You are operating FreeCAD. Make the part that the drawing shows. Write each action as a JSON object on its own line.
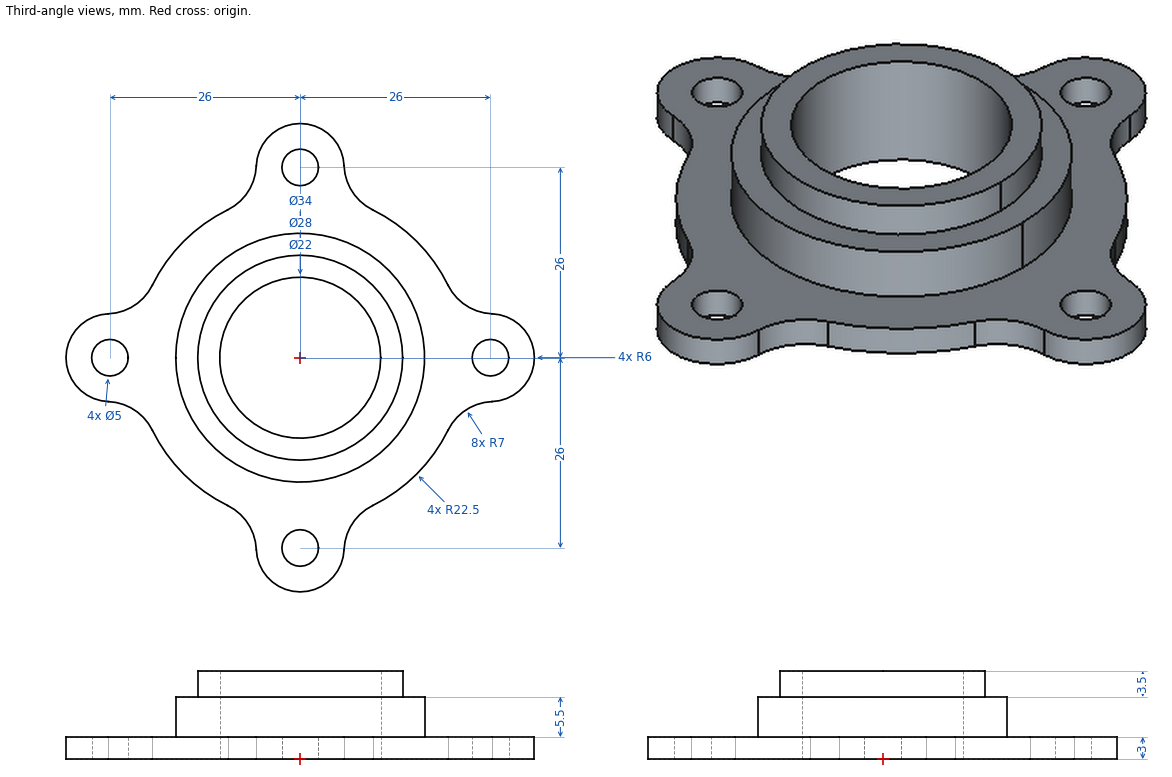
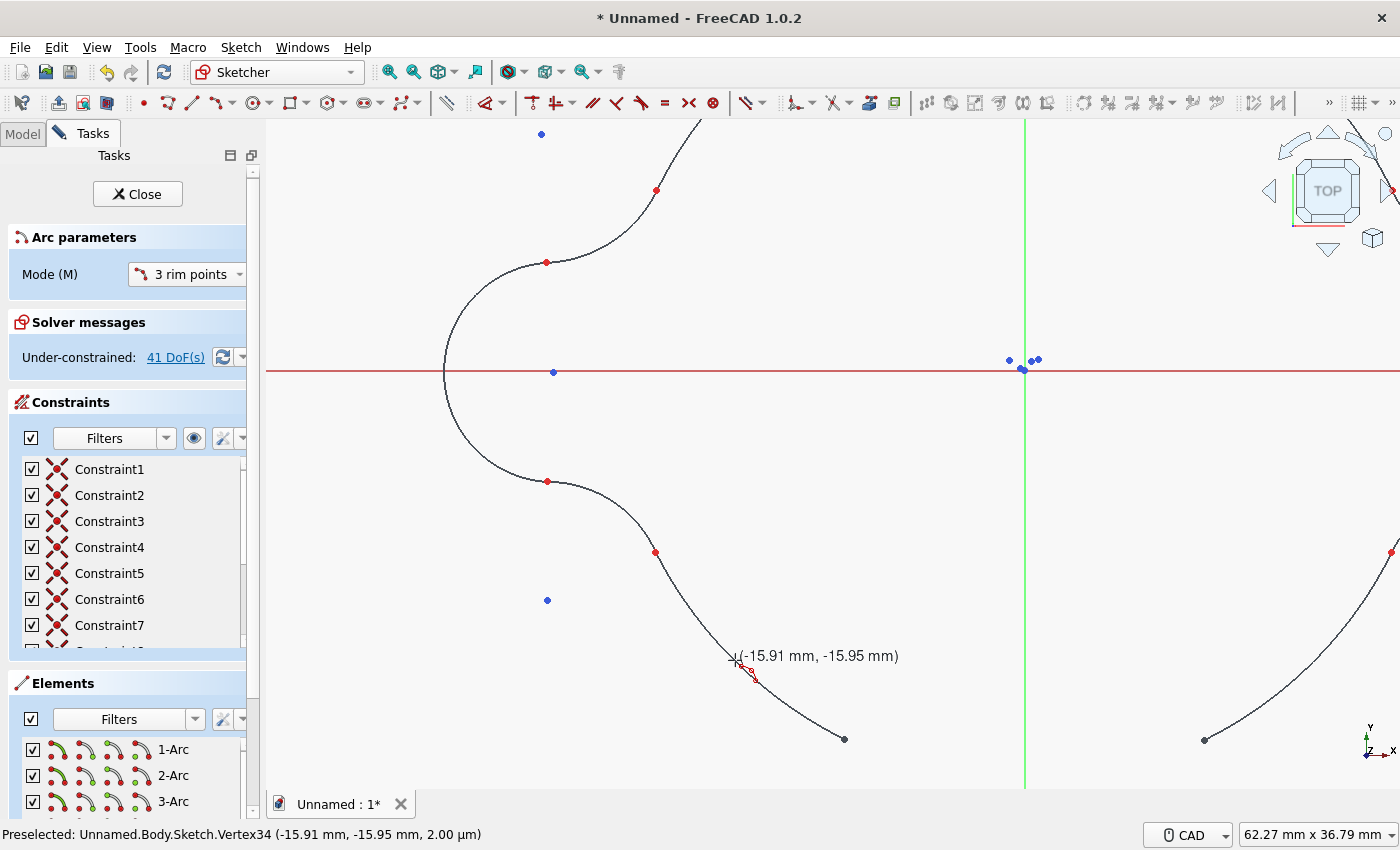
{"action": "left_click", "coordinate": [844, 739]}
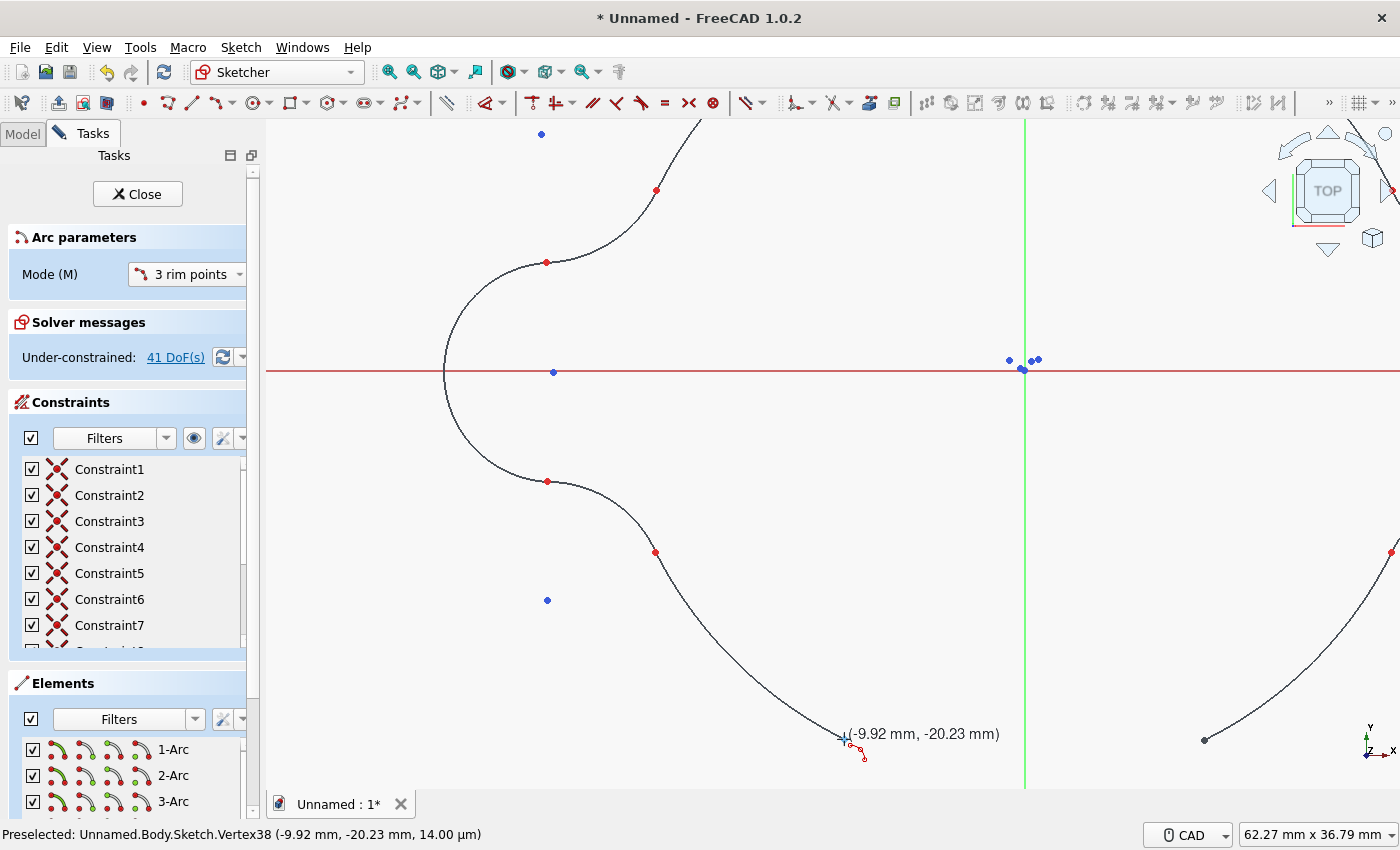
{"action": "scroll", "coordinate": [613, 503], "scroll_direction": "down", "scroll_amount": 5}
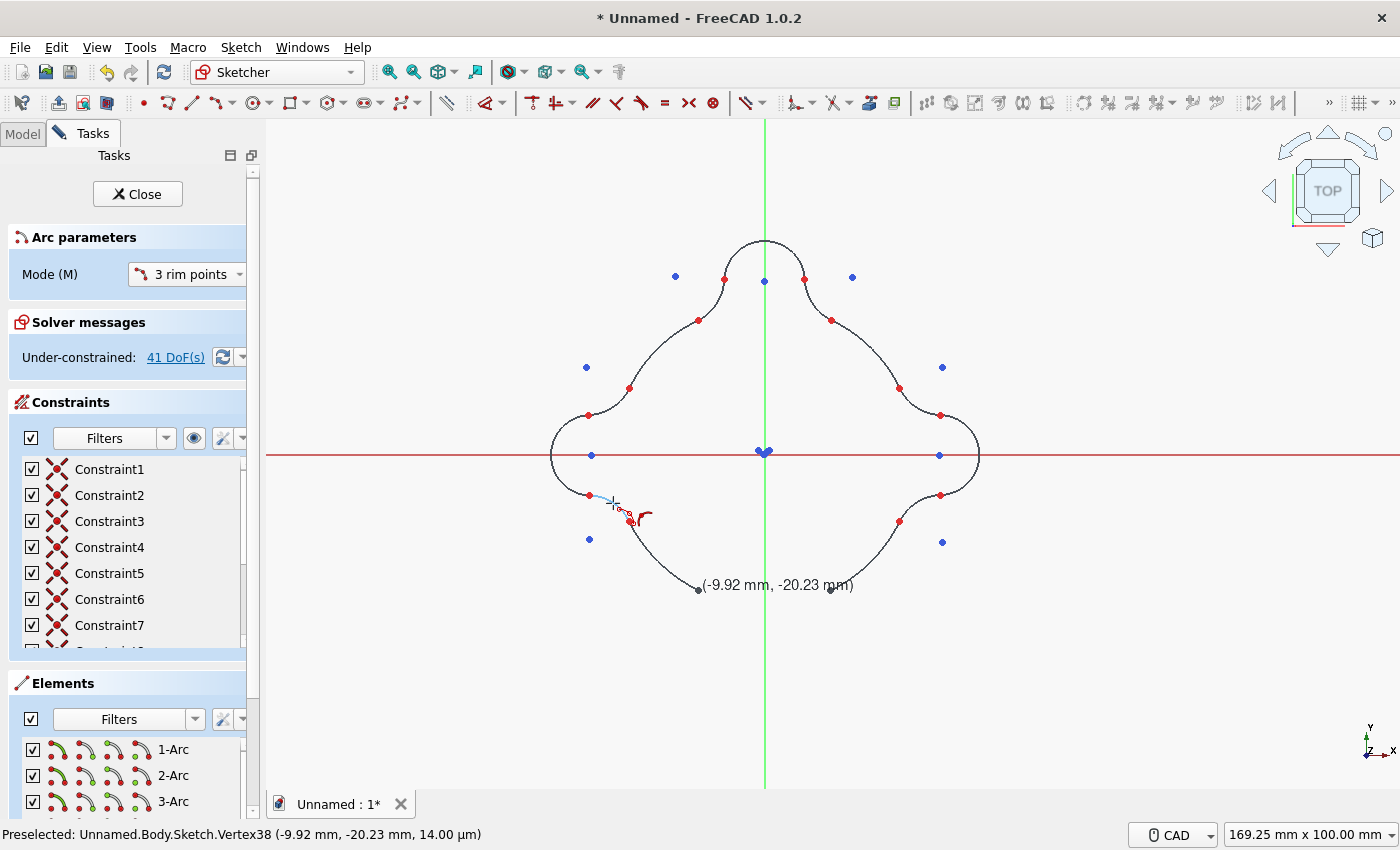
{"action": "left_click", "coordinate": [724, 630]}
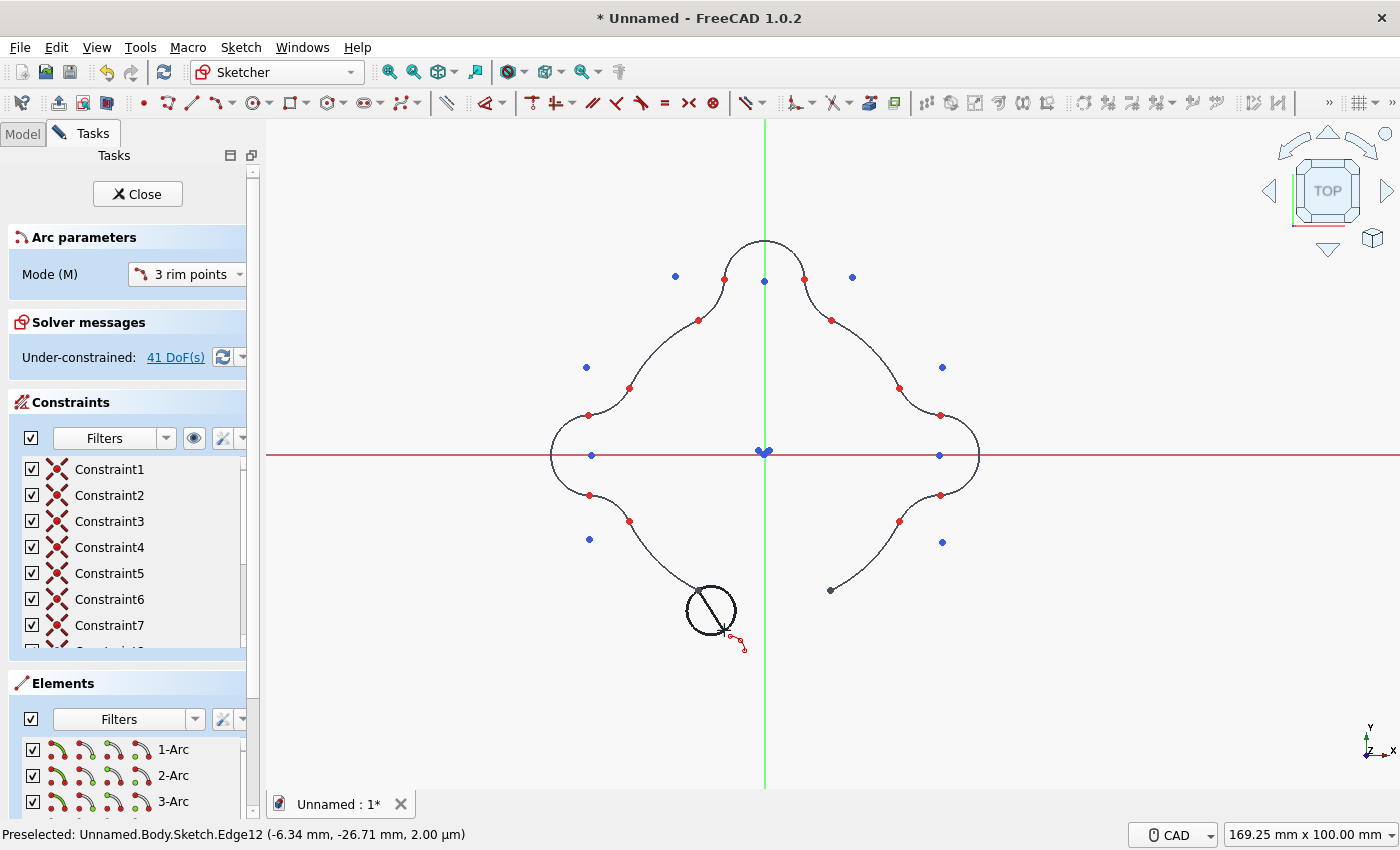
{"action": "scroll", "coordinate": [717, 607], "scroll_direction": "up", "scroll_amount": 5}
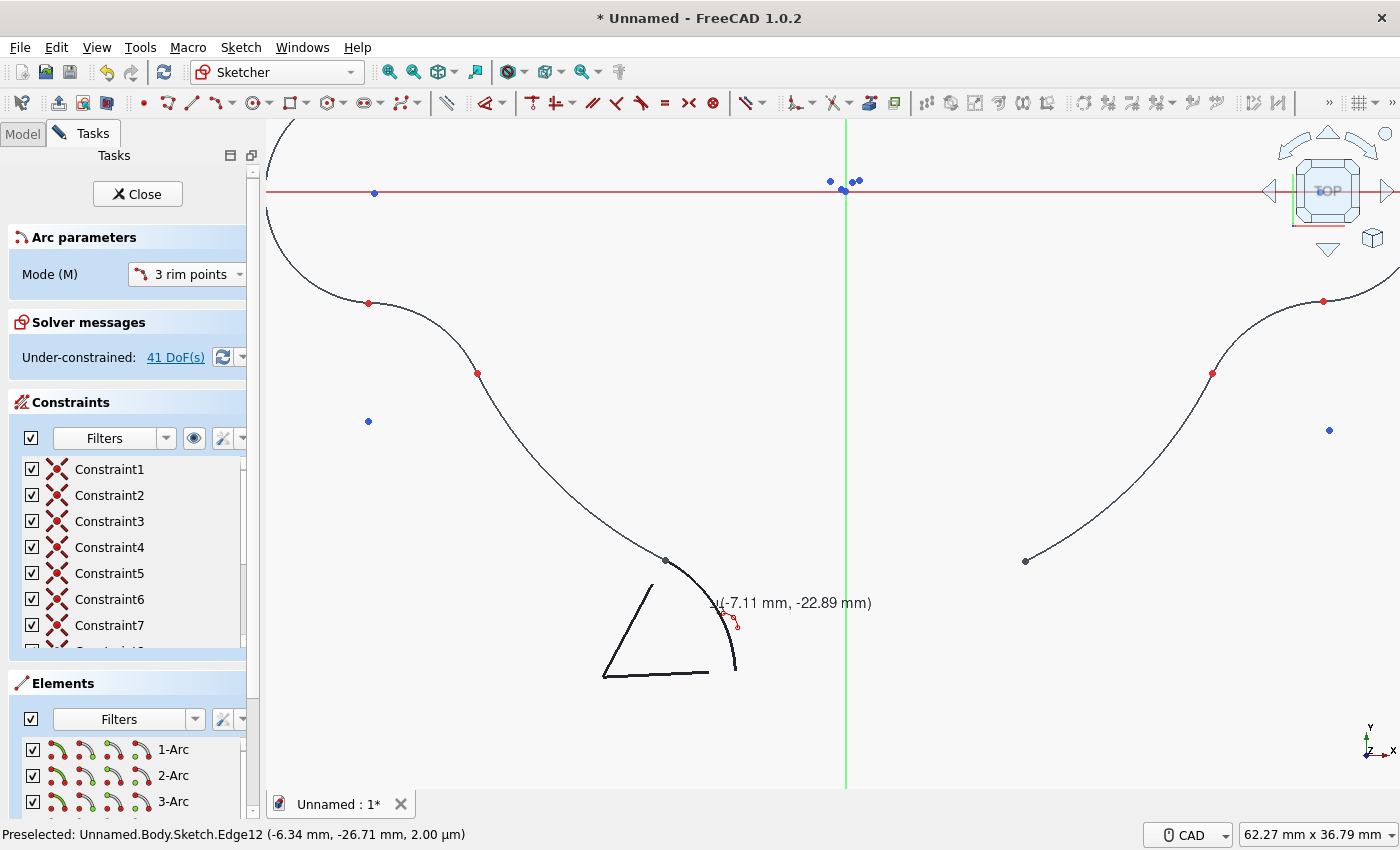
{"action": "left_click", "coordinate": [716, 604]}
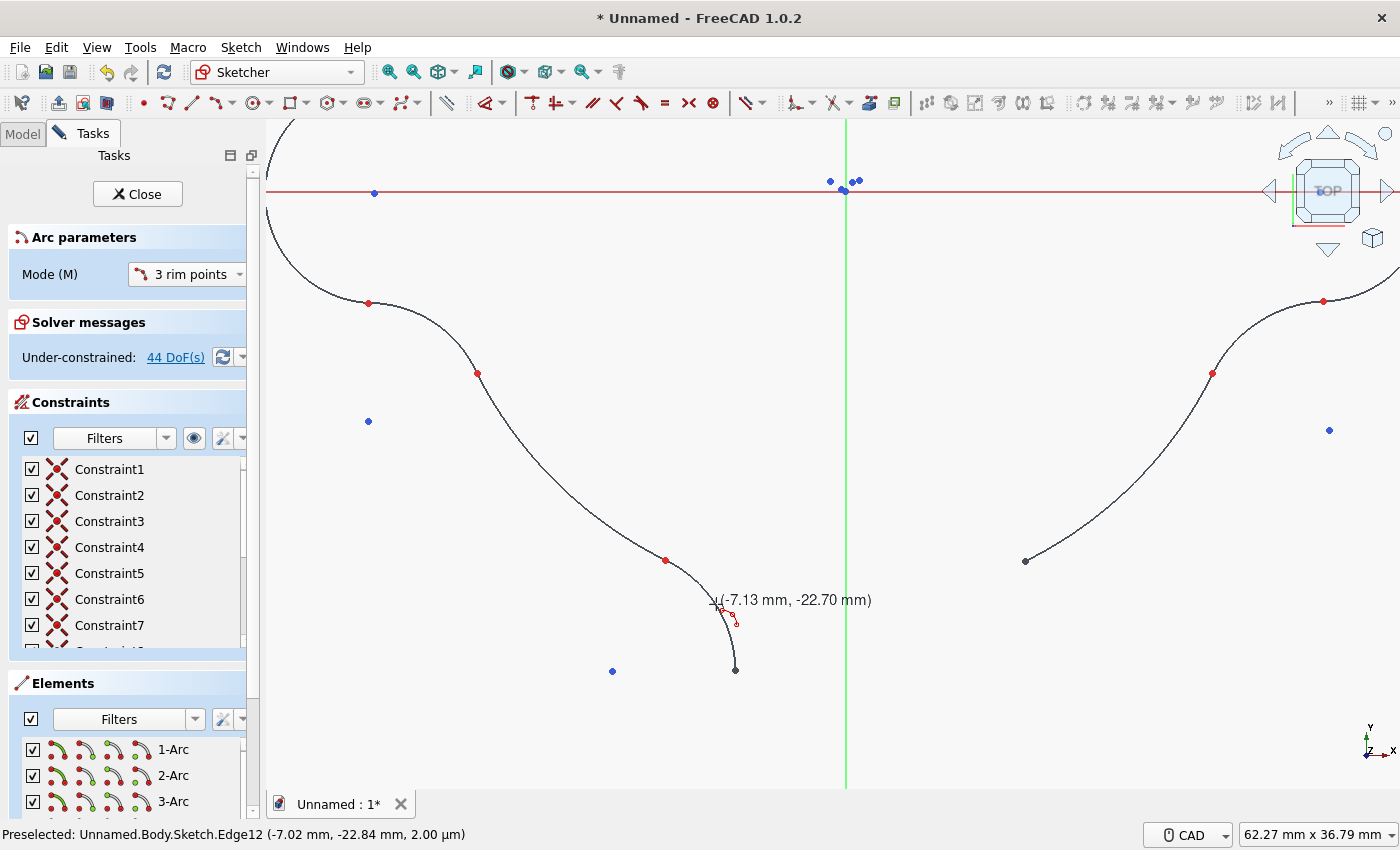
{"action": "left_click", "coordinate": [735, 671]}
{"action": "left_click", "coordinate": [955, 669]}
{"action": "left_click", "coordinate": [783, 754]}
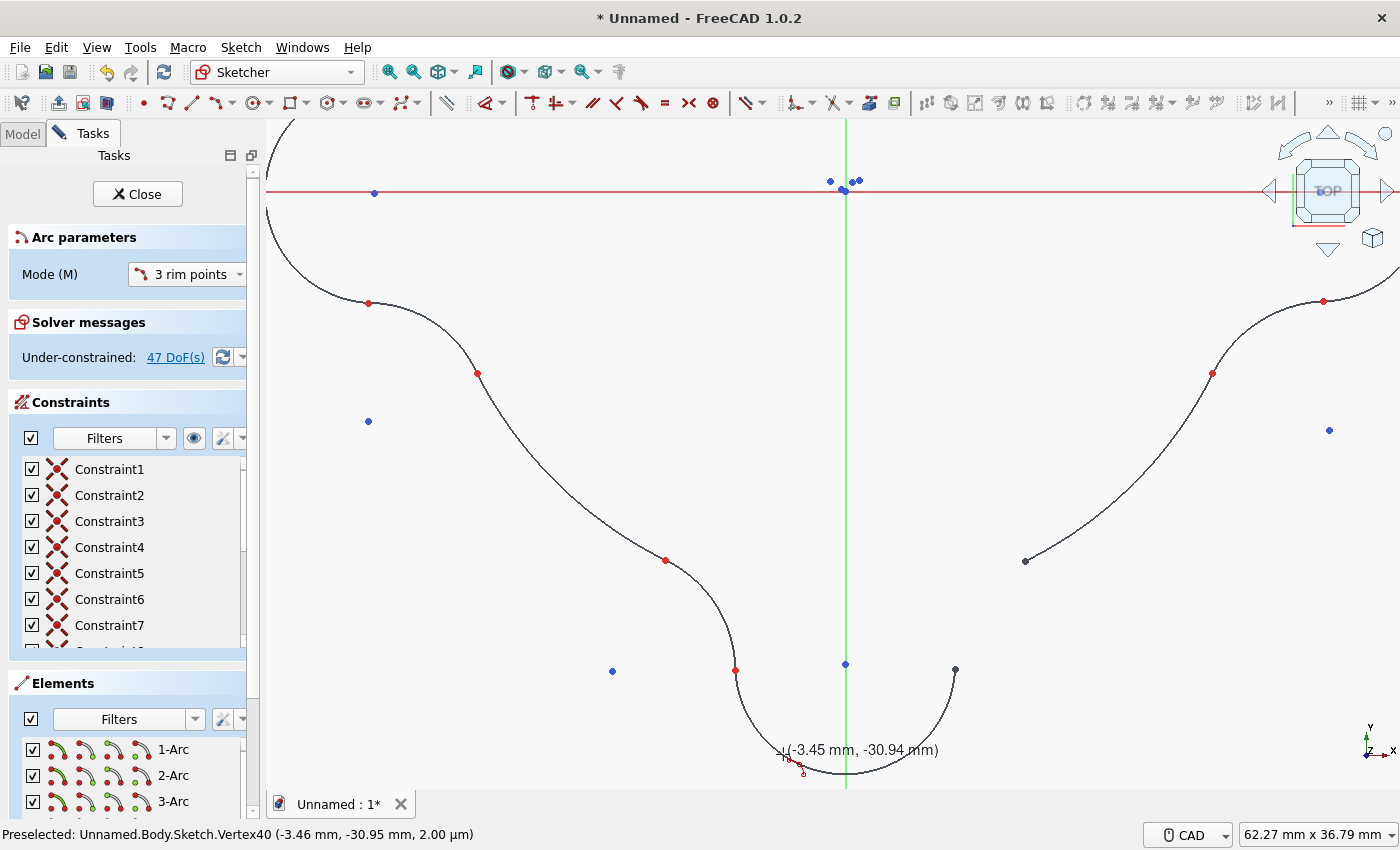
{"action": "left_click", "coordinate": [955, 670]}
{"action": "left_click", "coordinate": [1025, 561]}
{"action": "left_click", "coordinate": [976, 604]}
{"action": "key", "text": "Escape"}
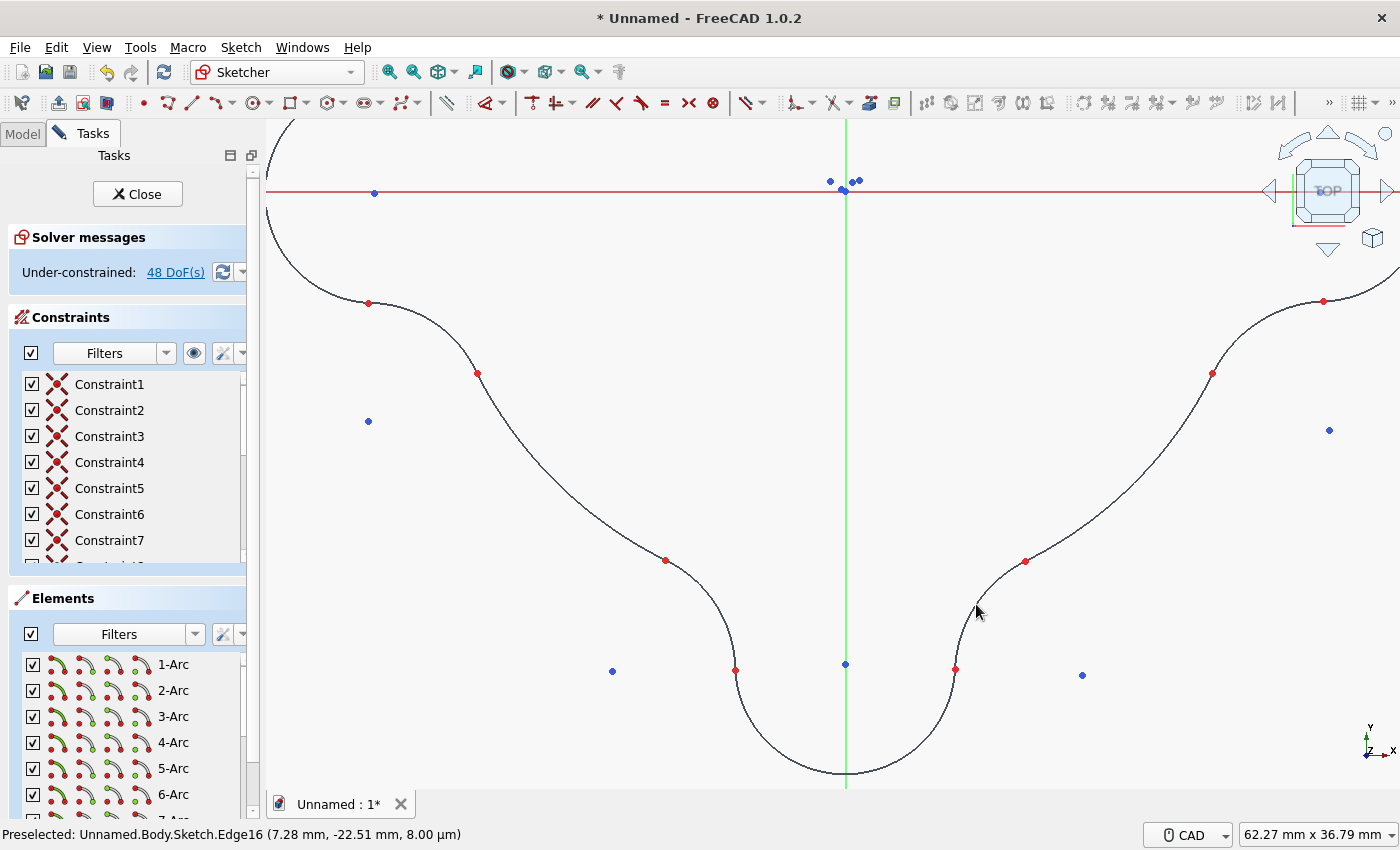
{"action": "left_click", "coordinate": [1094, 518]}